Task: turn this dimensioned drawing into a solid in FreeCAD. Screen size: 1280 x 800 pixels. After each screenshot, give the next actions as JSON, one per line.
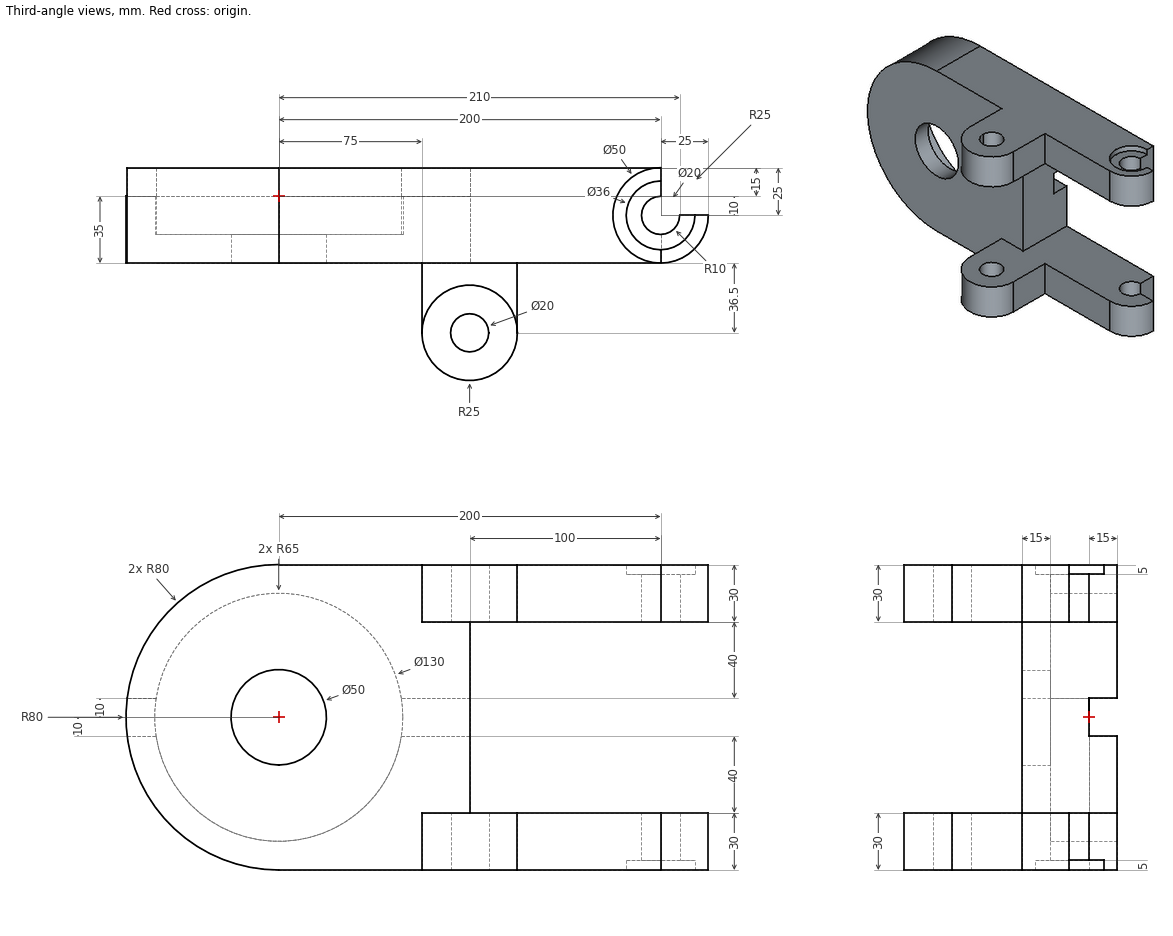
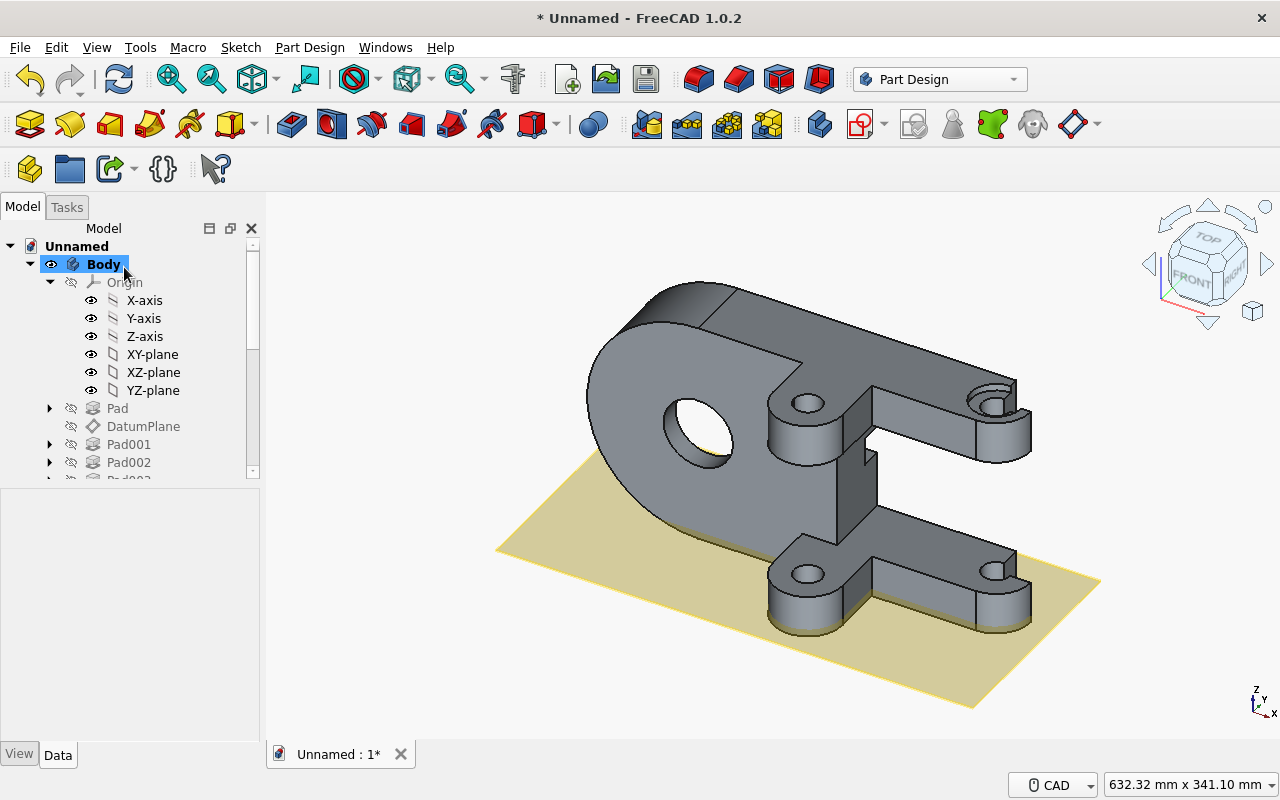
{"action": "scroll", "coordinate": [100, 350], "scroll_direction": "down", "scroll_amount": 3}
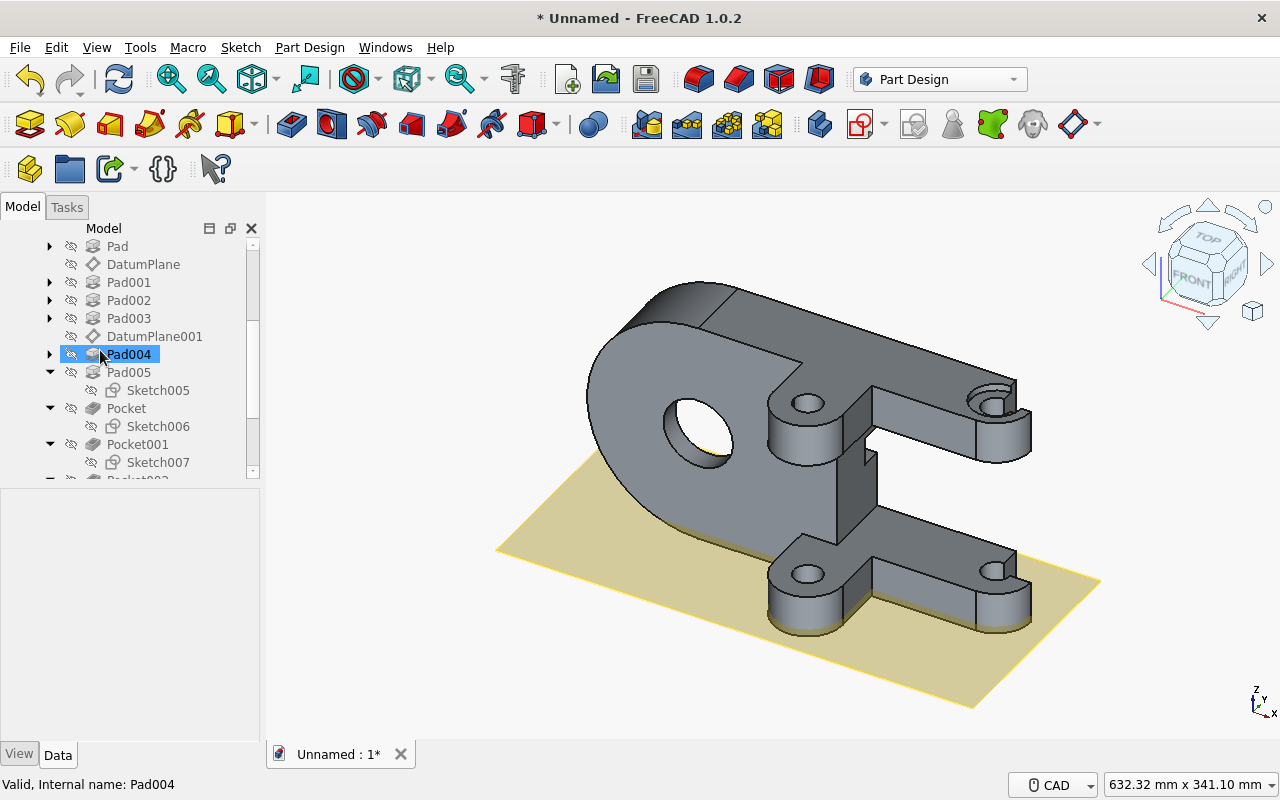
{"action": "scroll", "coordinate": [140, 350], "scroll_direction": "up", "scroll_amount": 15}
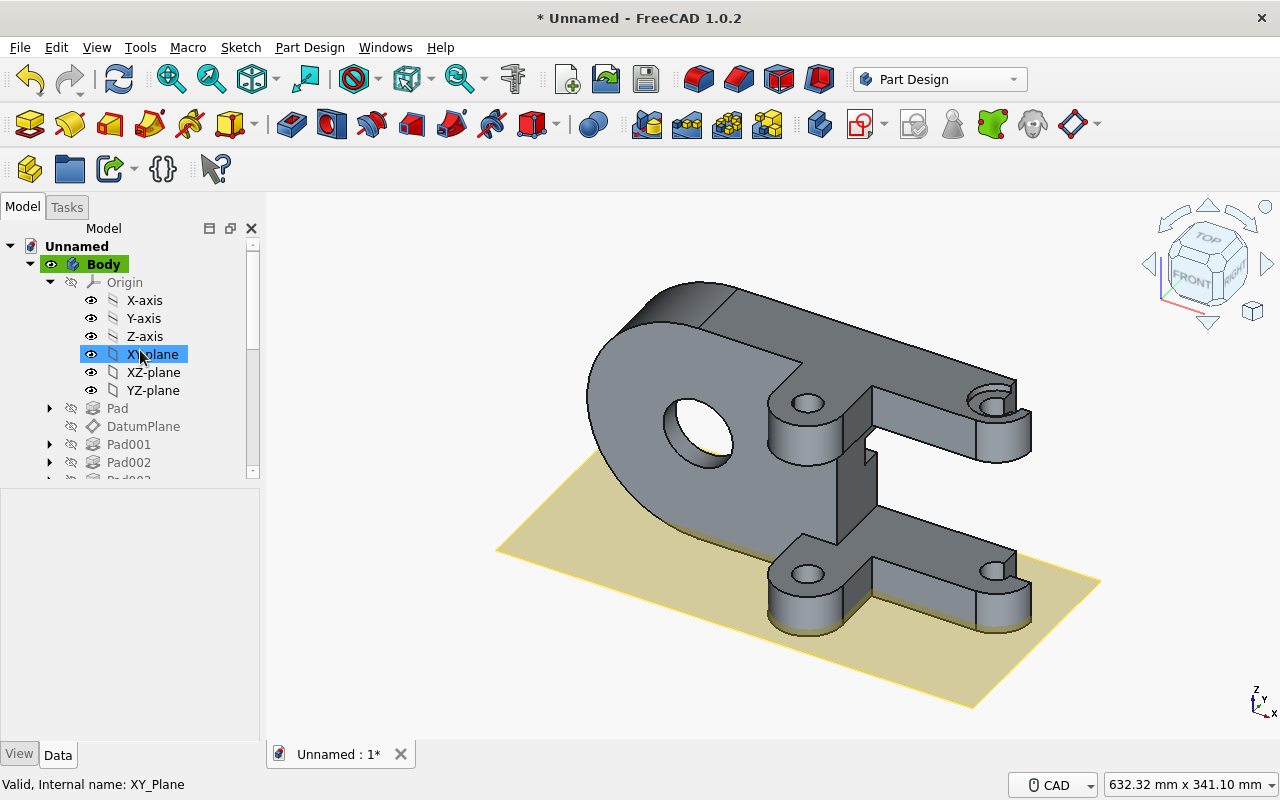
{"action": "scroll", "coordinate": [100, 350], "scroll_direction": "down", "scroll_amount": 6}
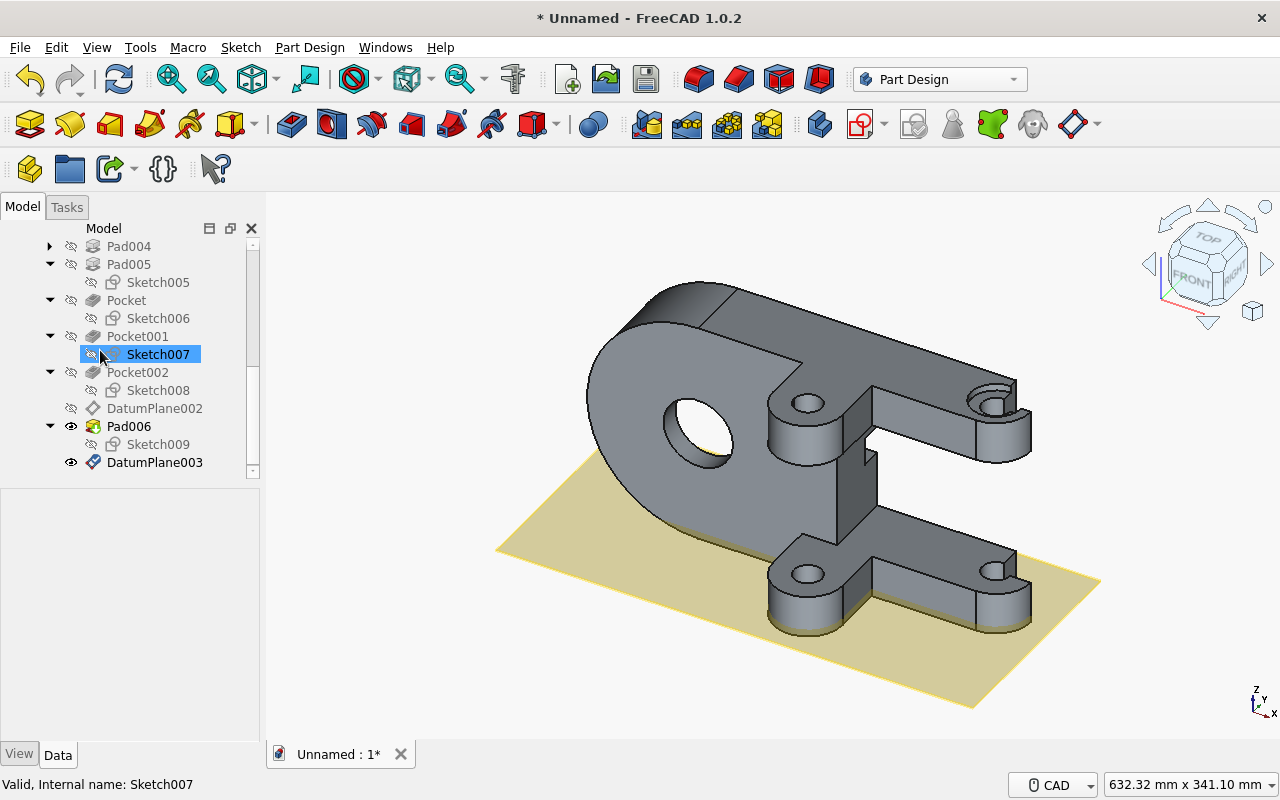
{"action": "left_click", "coordinate": [116, 462]}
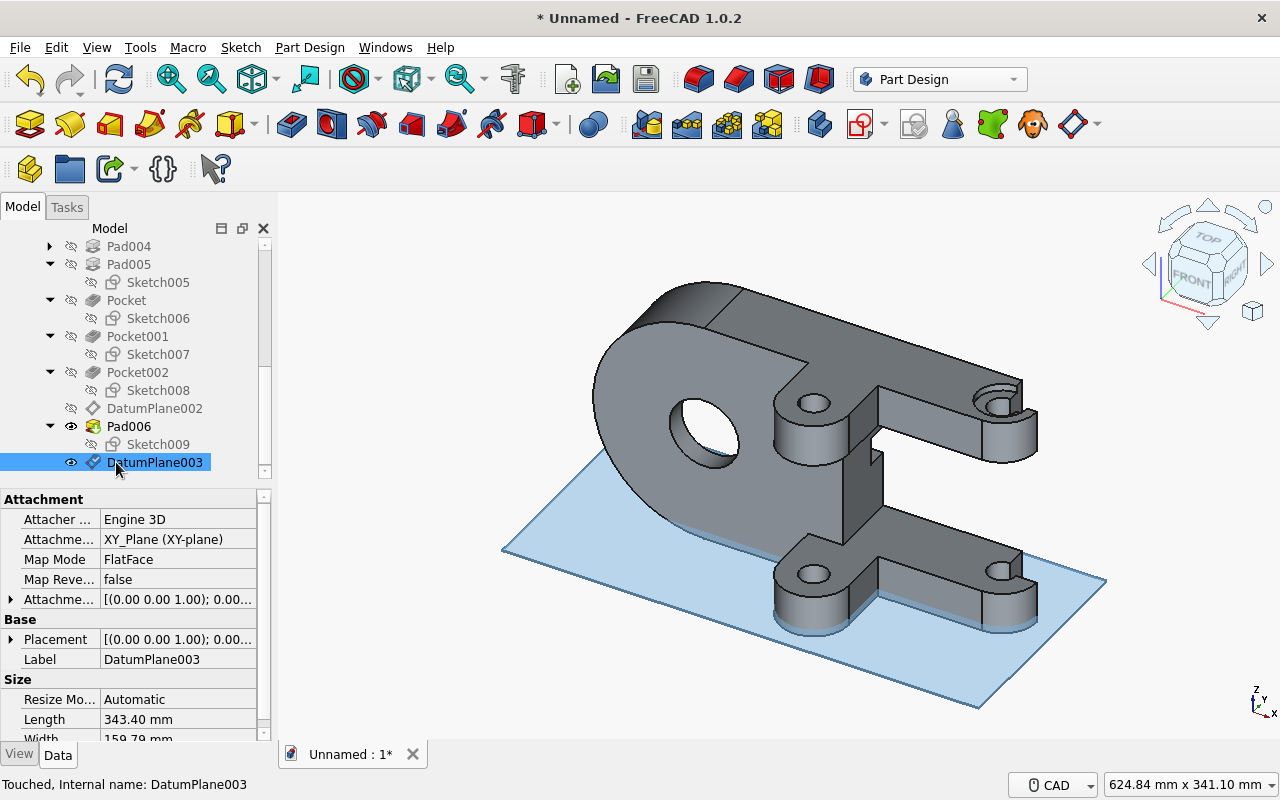
{"action": "left_click", "coordinate": [860, 124]}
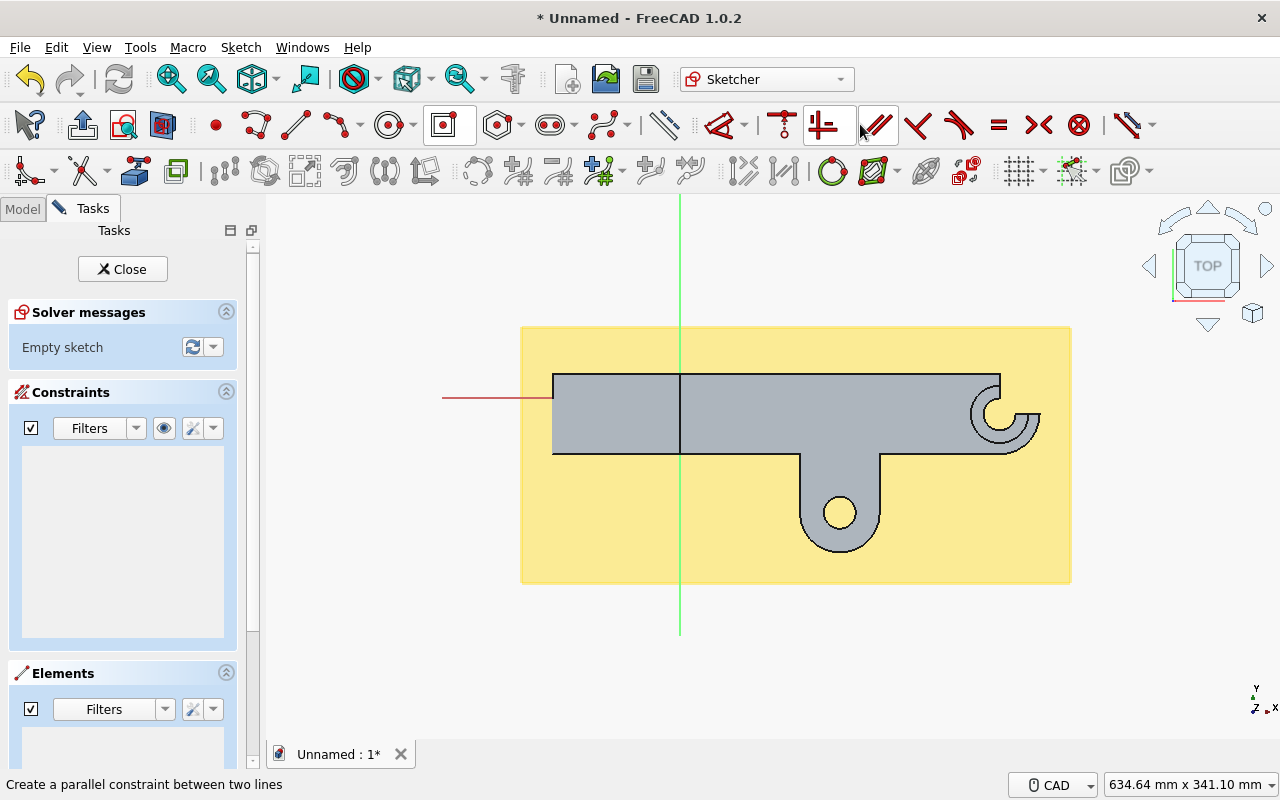
{"action": "left_click", "coordinate": [164, 126]}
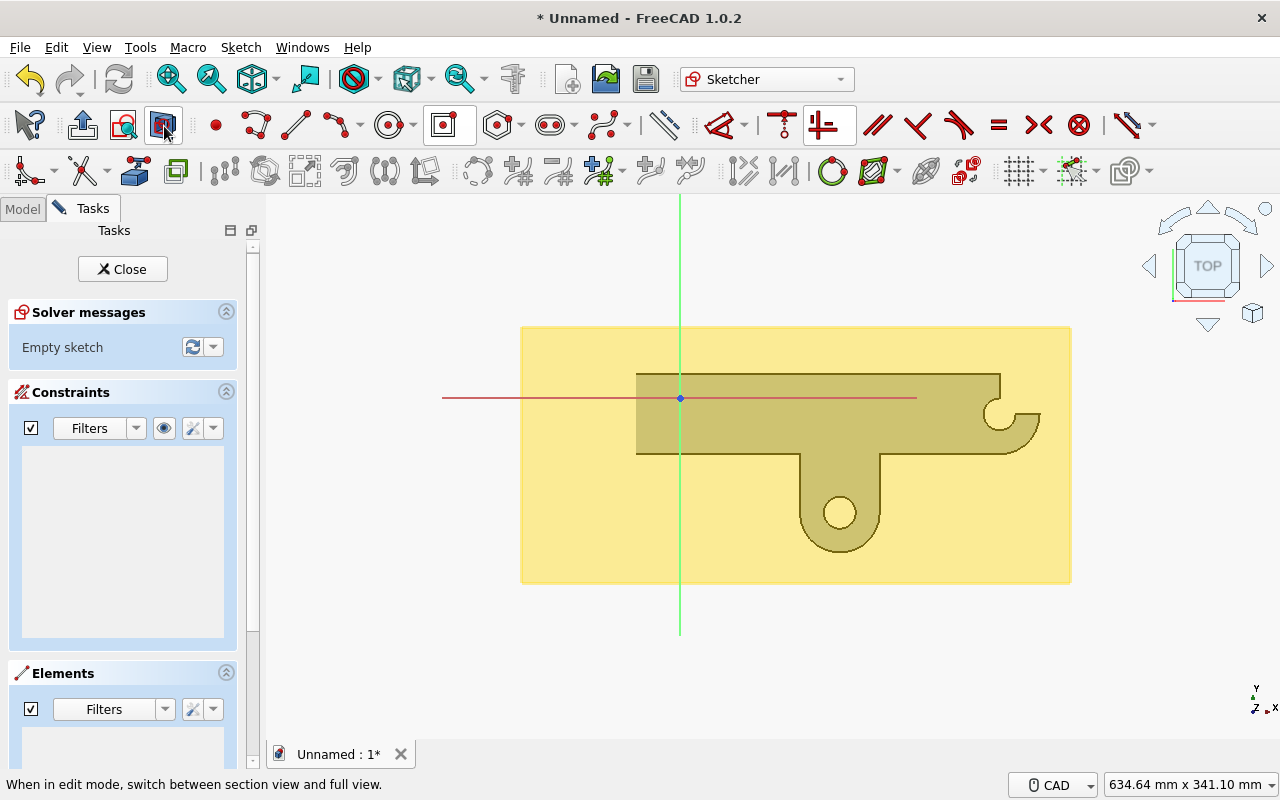
{"action": "scroll", "coordinate": [1058, 404], "scroll_direction": "up", "scroll_amount": 9}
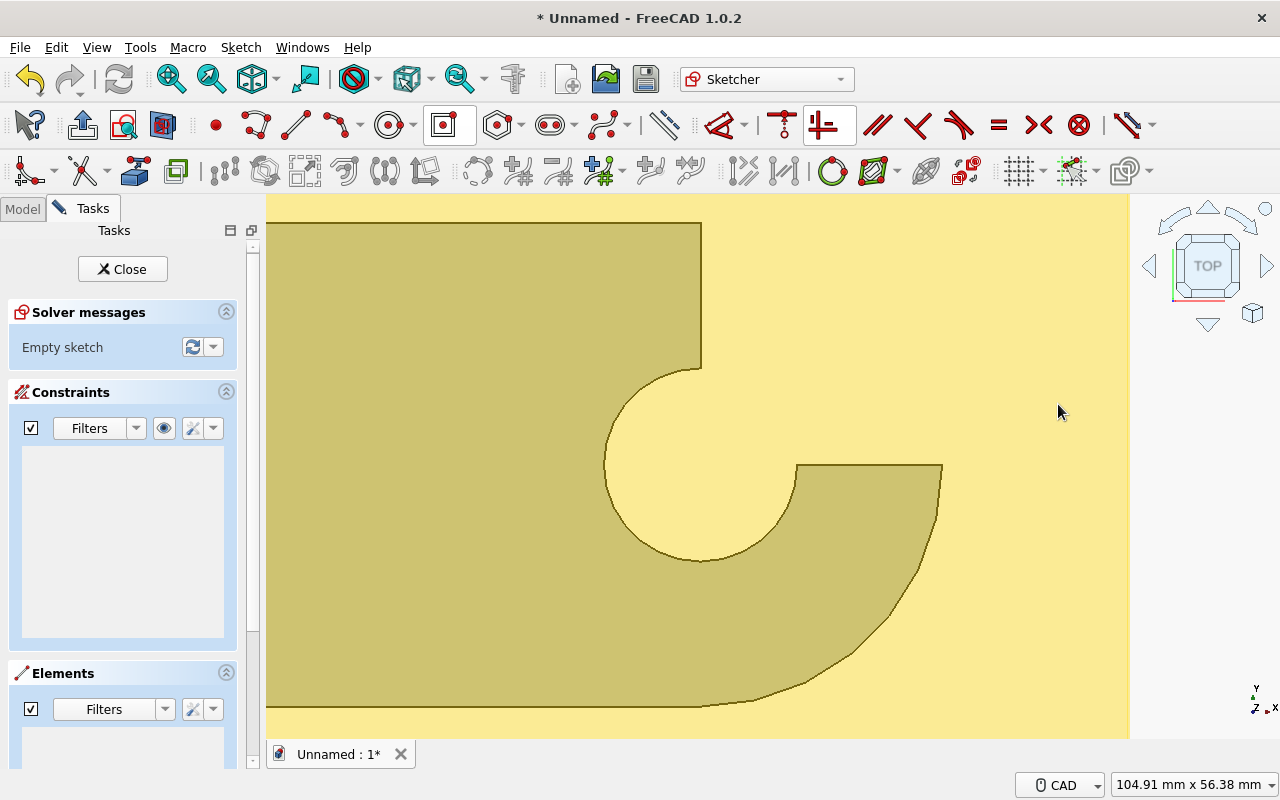
{"action": "left_click", "coordinate": [390, 126]}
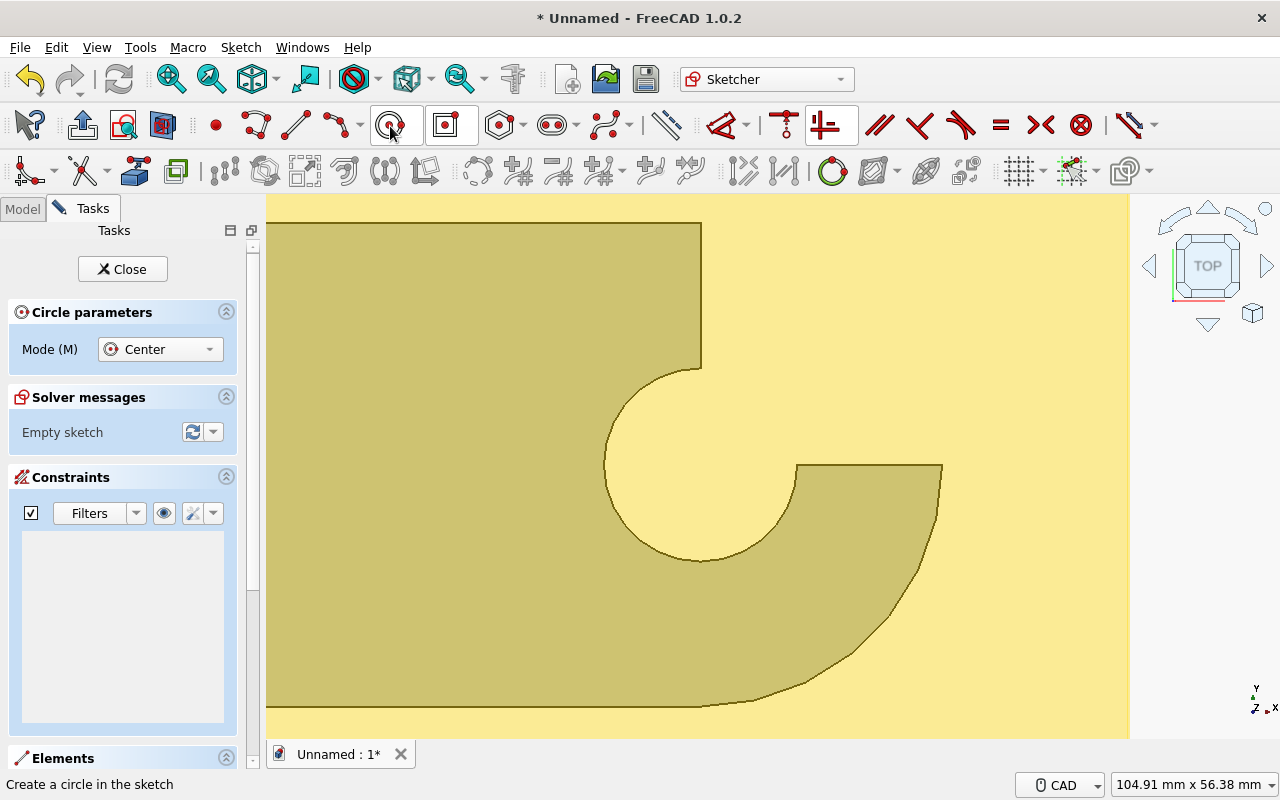
{"action": "left_click", "coordinate": [701, 465]}
{"action": "left_click", "coordinate": [824, 342]}
{"action": "key", "text": "Escape"}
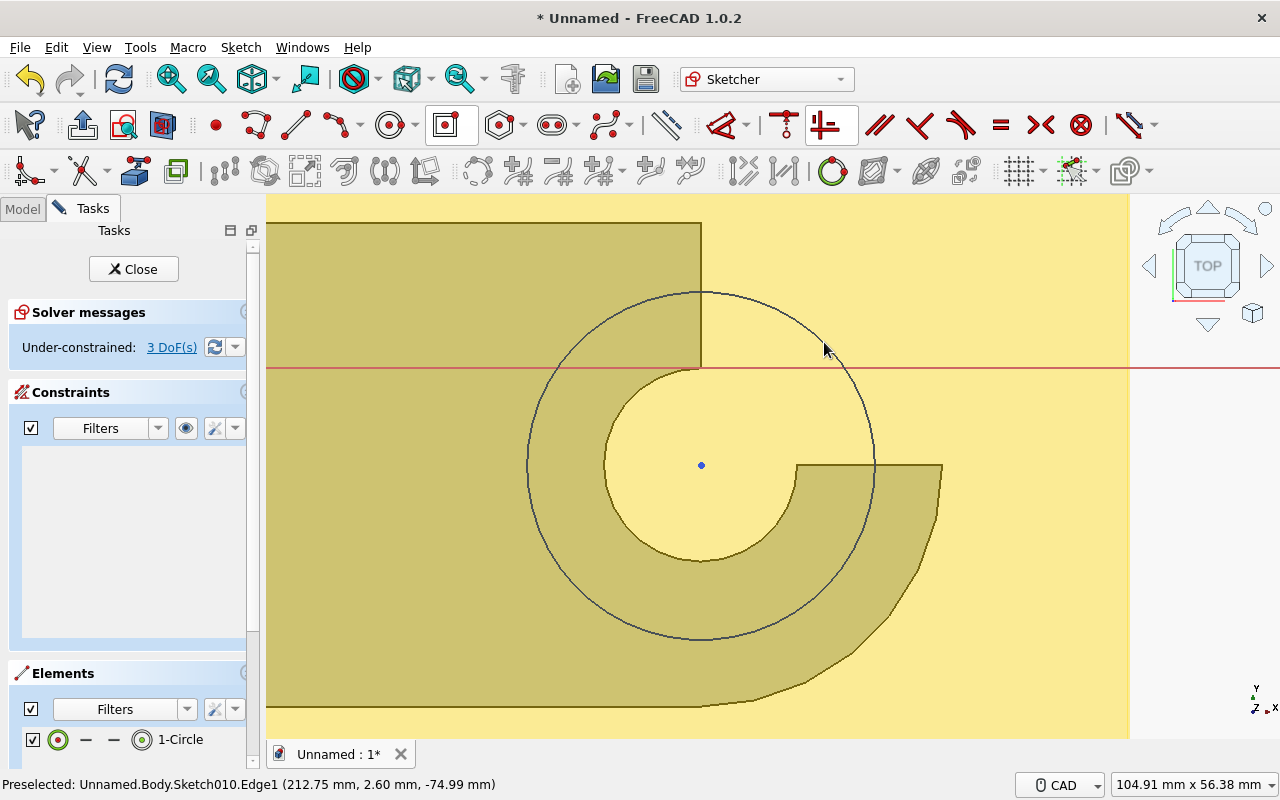
{"action": "left_click", "coordinate": [722, 126]}